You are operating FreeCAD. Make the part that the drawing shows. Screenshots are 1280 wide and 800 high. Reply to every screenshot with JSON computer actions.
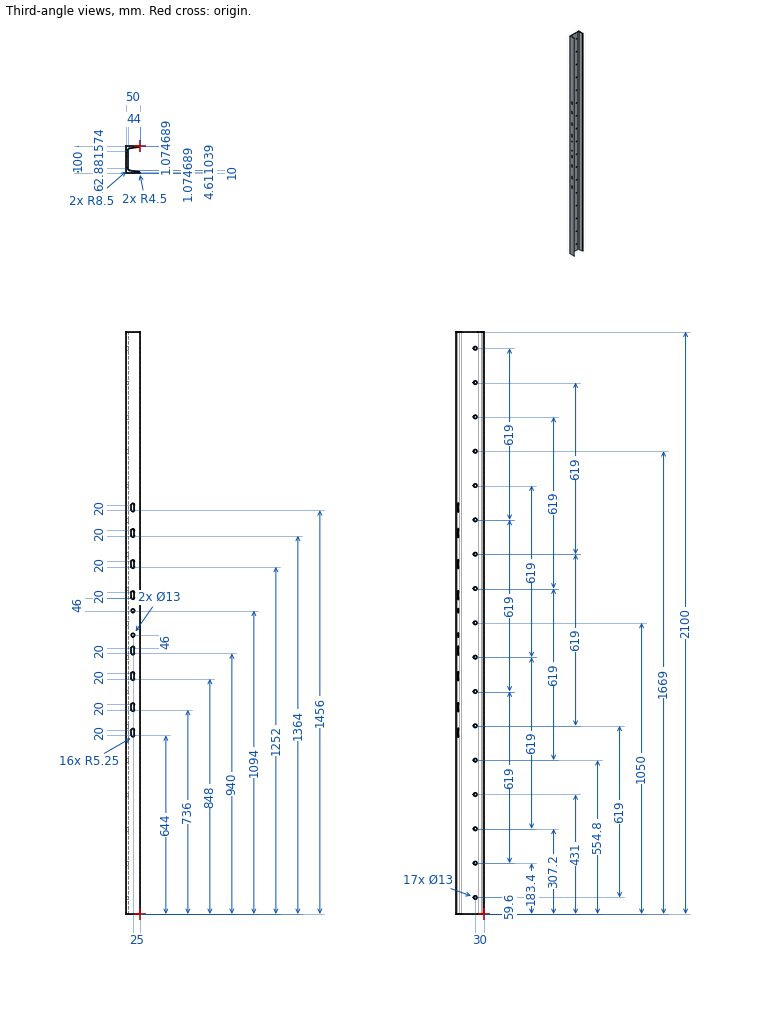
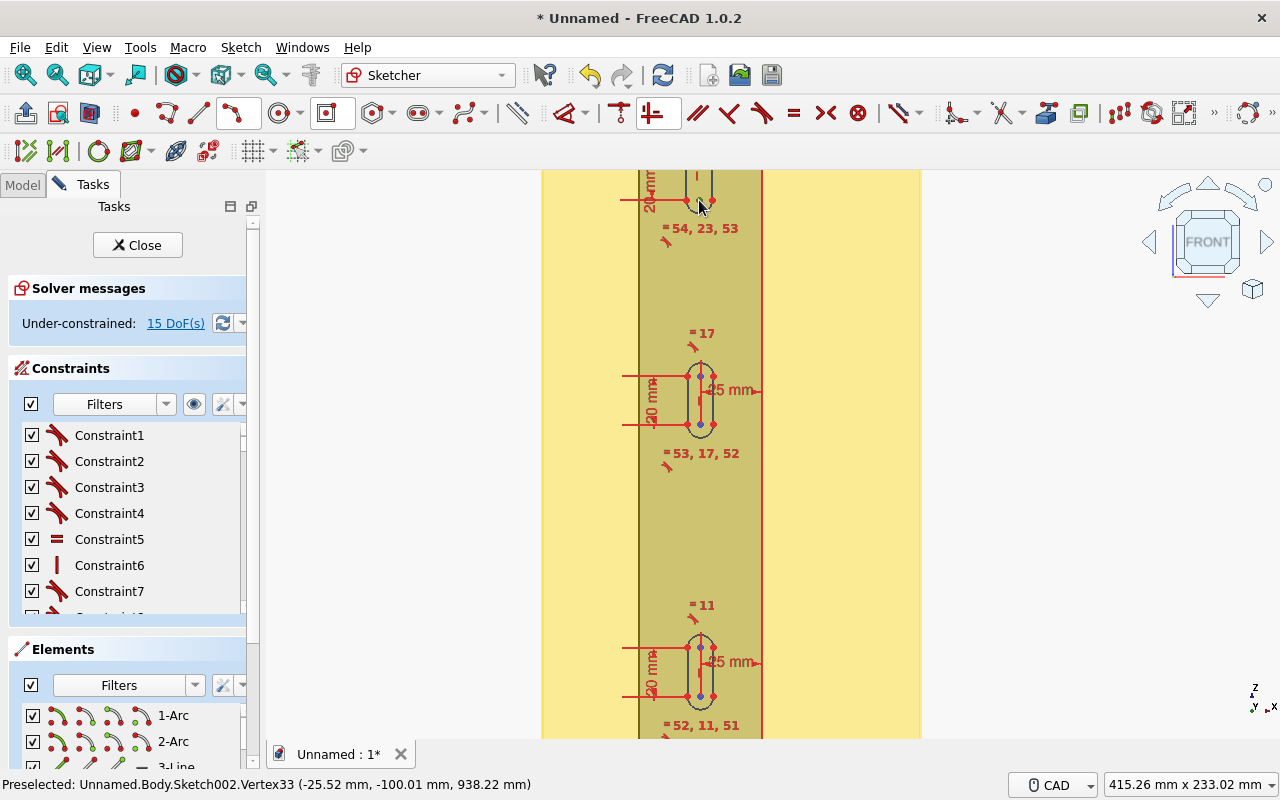
{"action": "left_click", "coordinate": [588, 114]}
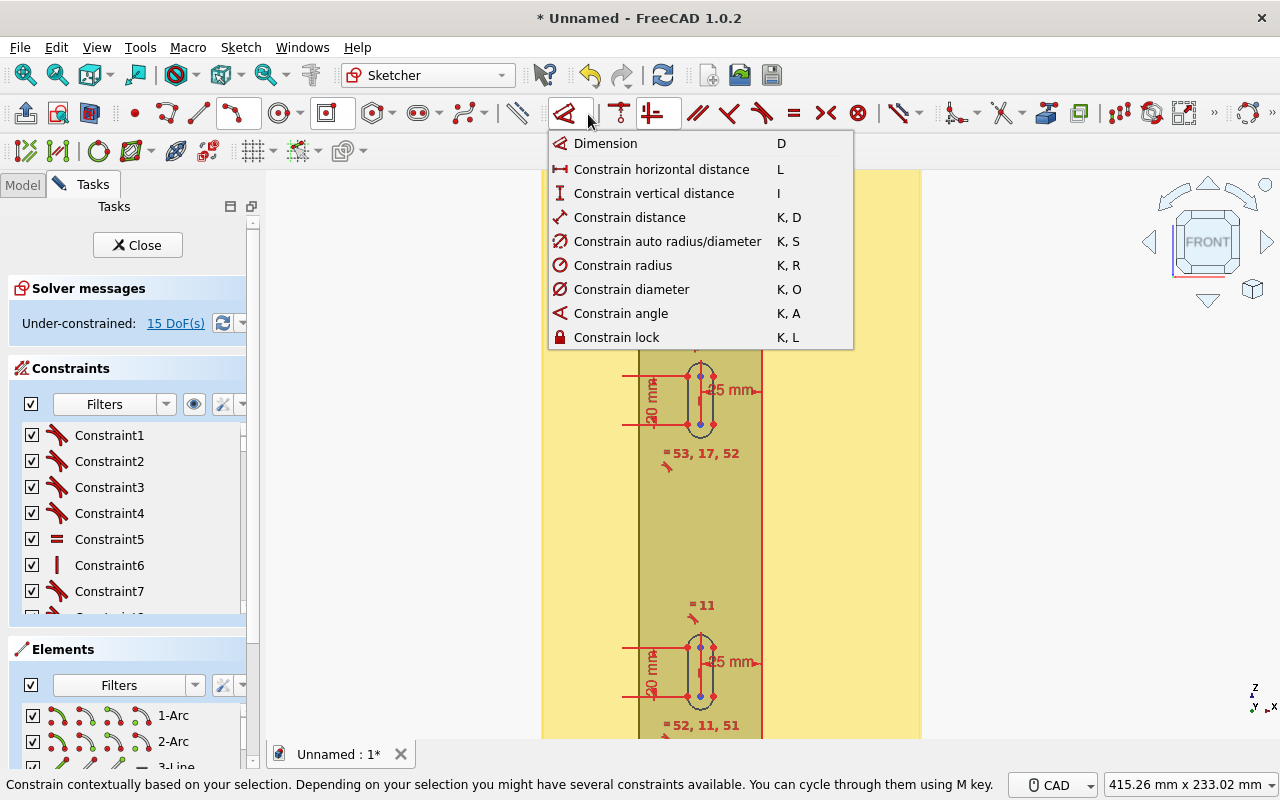
{"action": "left_click", "coordinate": [701, 169]}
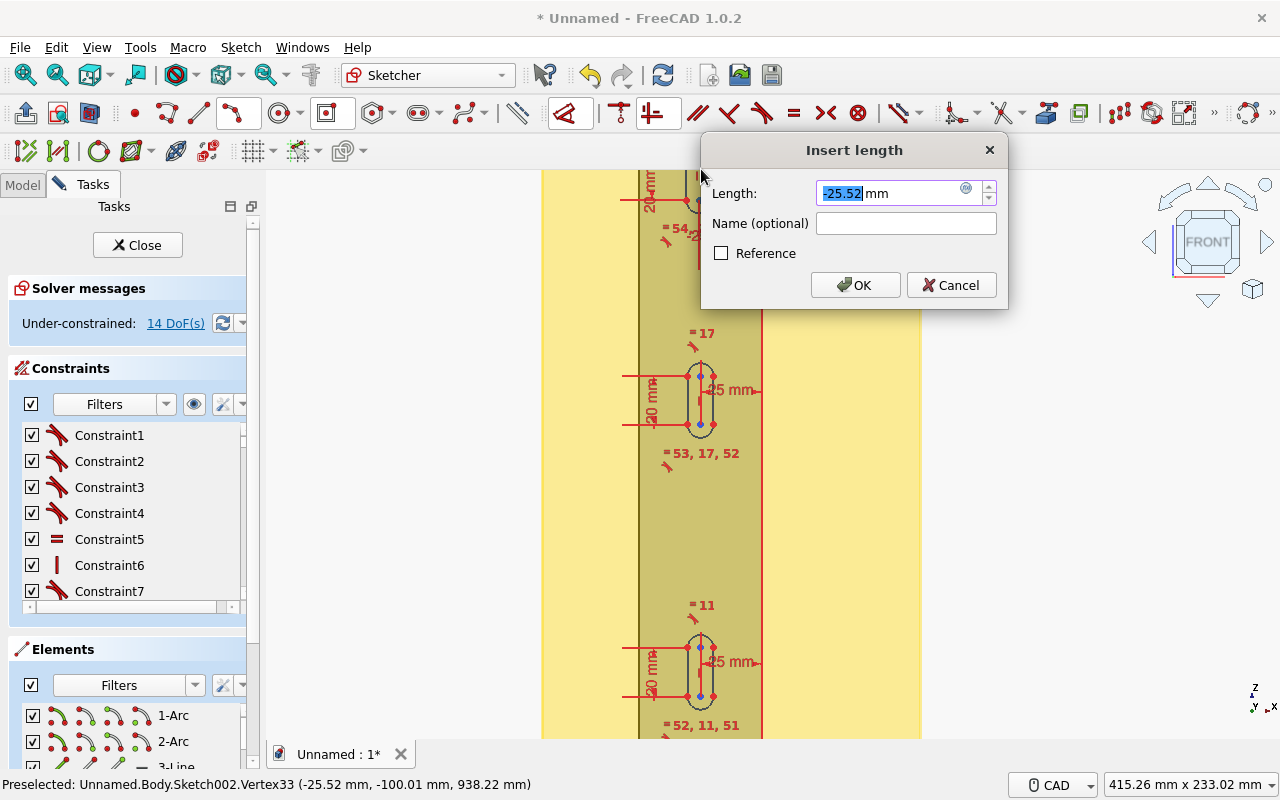
{"action": "type", "text": "-25"}
{"action": "key", "text": "Return"}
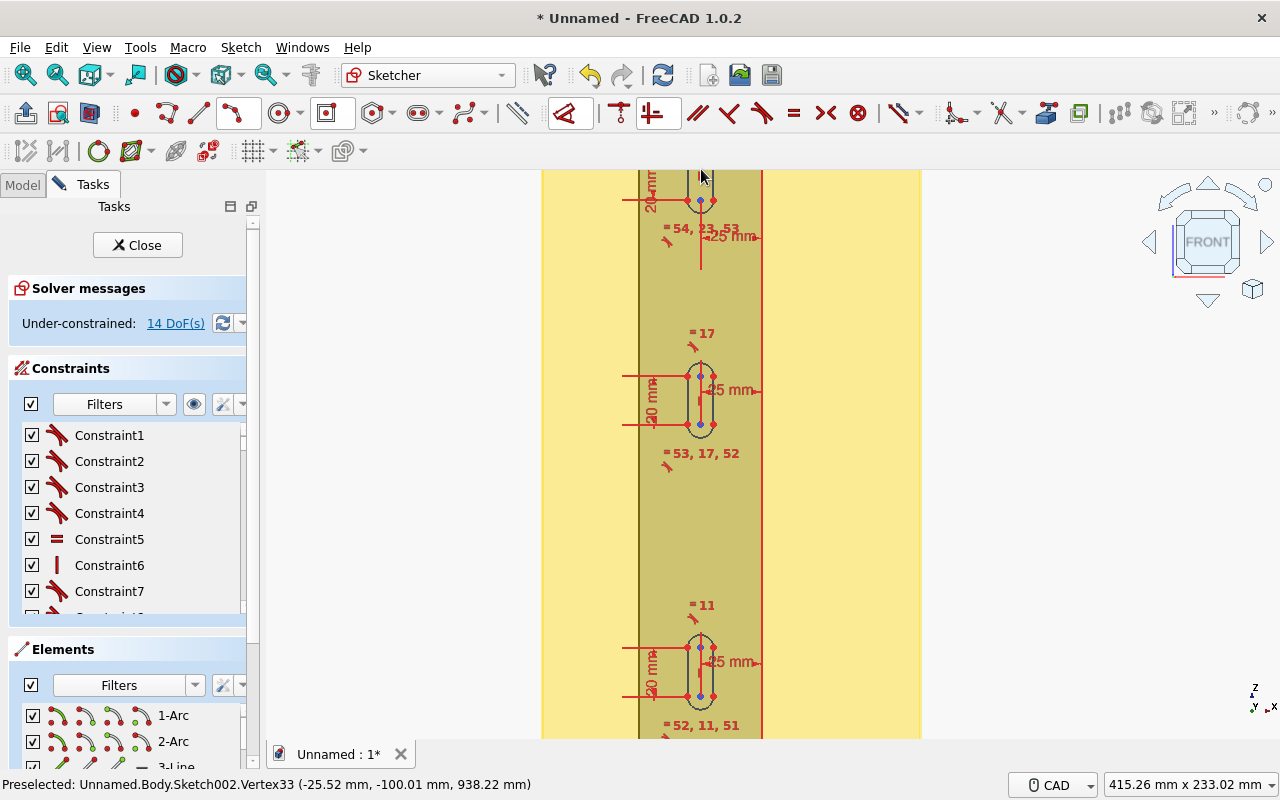
{"action": "scroll", "coordinate": [703, 432], "scroll_direction": "down", "scroll_amount": 12}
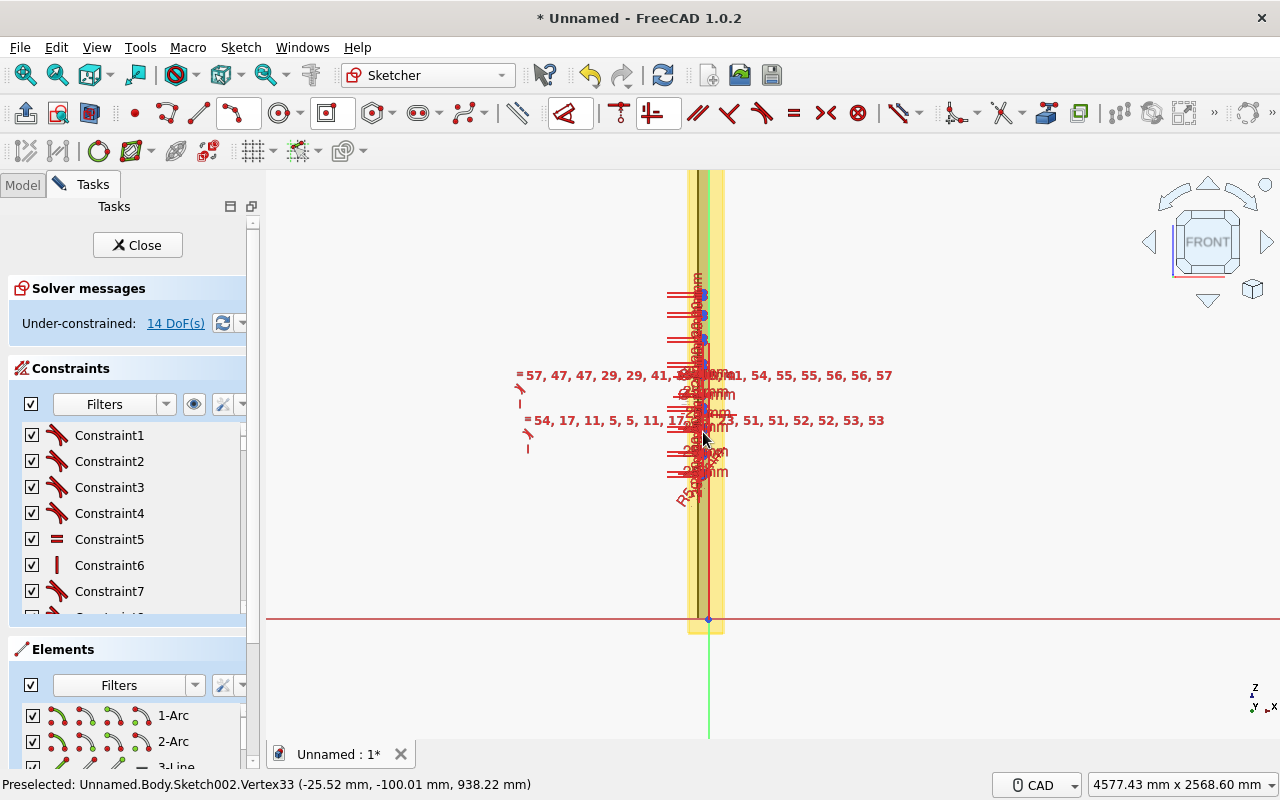
{"action": "scroll", "coordinate": [703, 342], "scroll_direction": "up", "scroll_amount": 12}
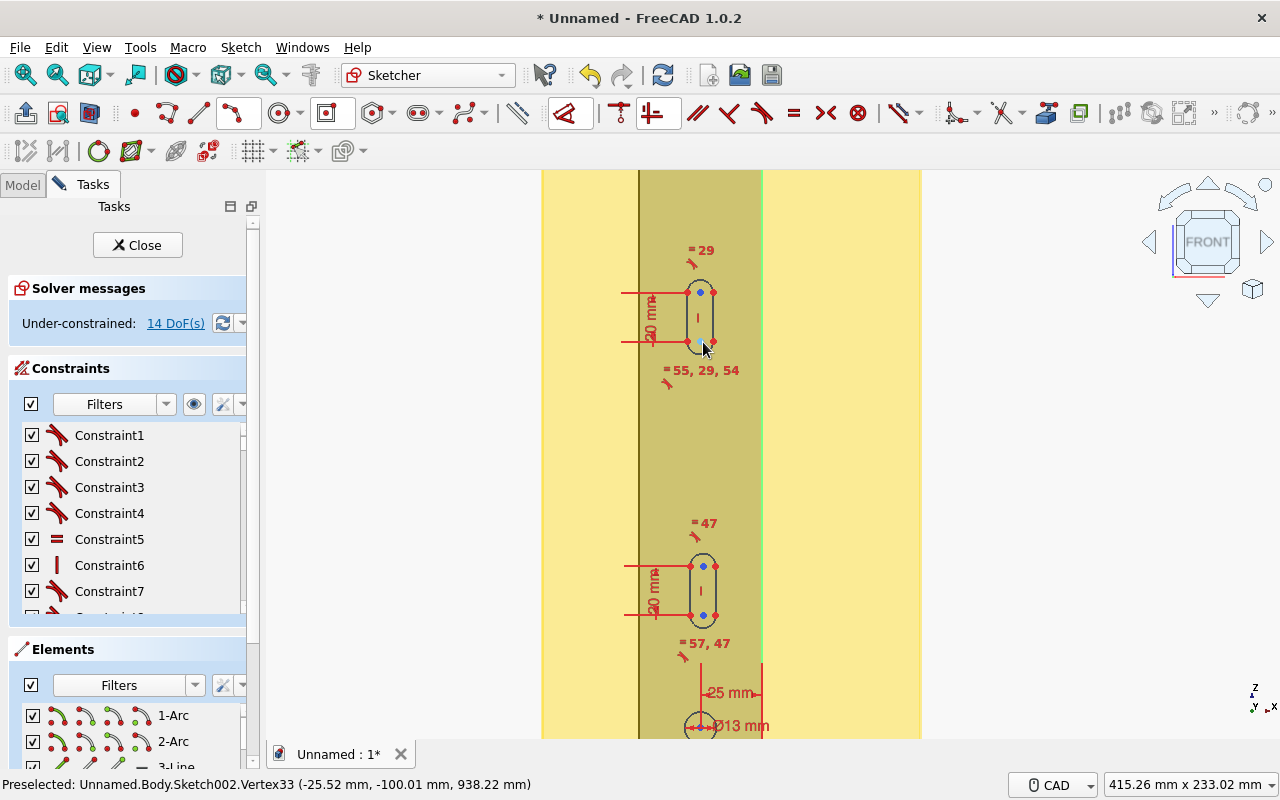
{"action": "left_click", "coordinate": [700, 342]}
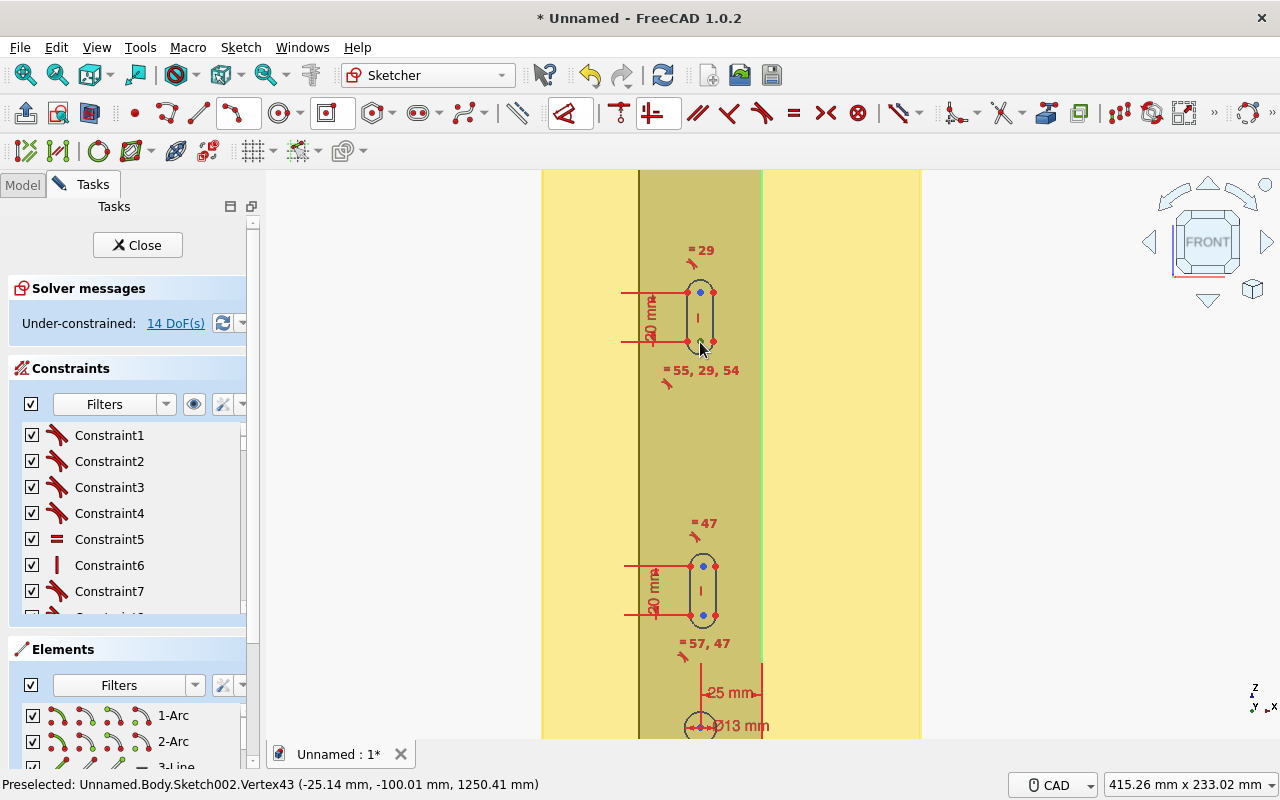
{"action": "left_click", "coordinate": [588, 114]}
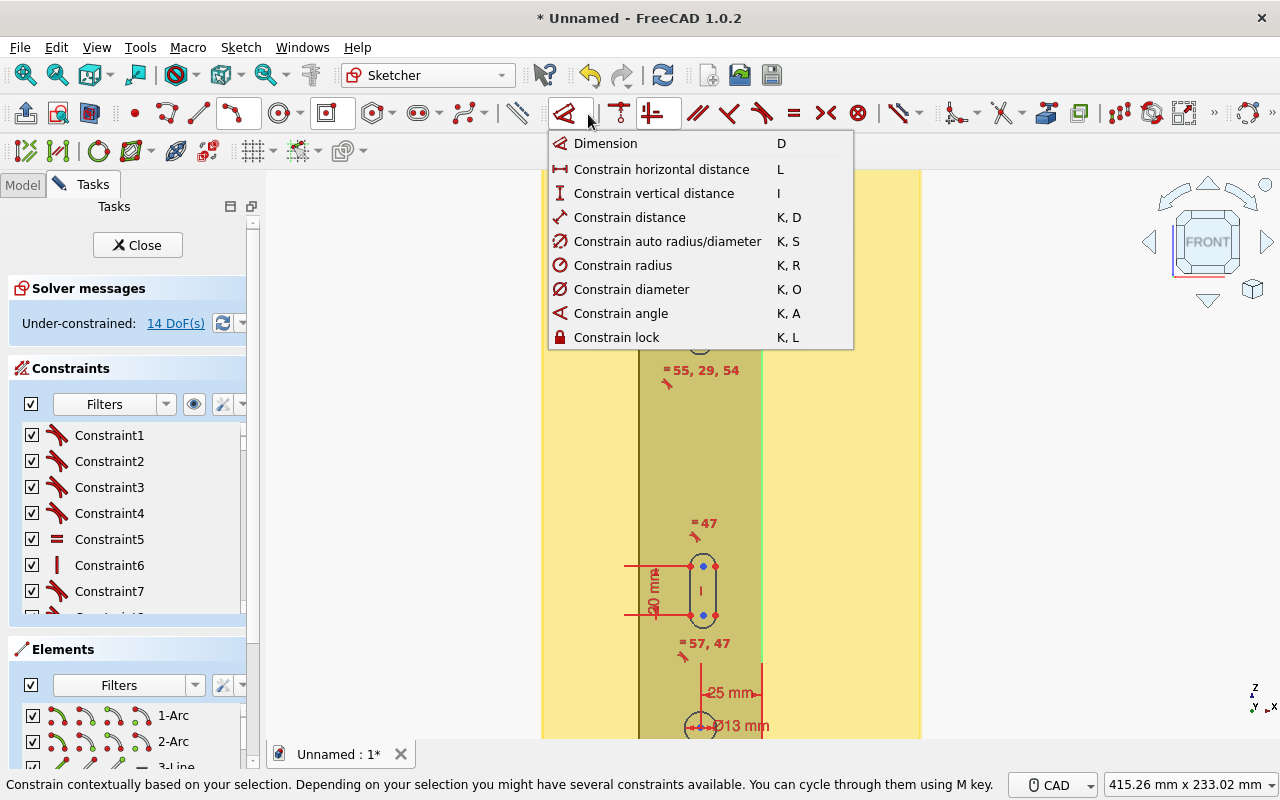
{"action": "left_click", "coordinate": [701, 169]}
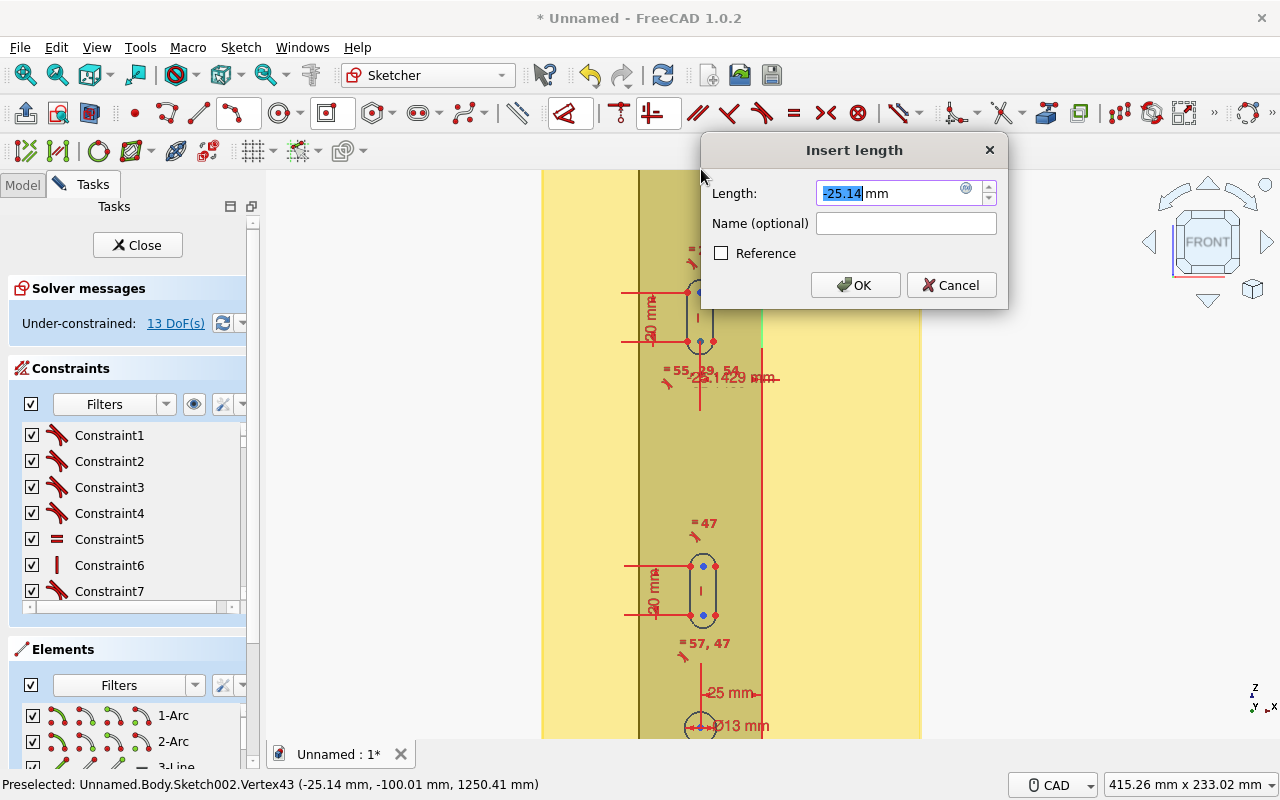
{"action": "type", "text": "-25"}
{"action": "key", "text": "Return"}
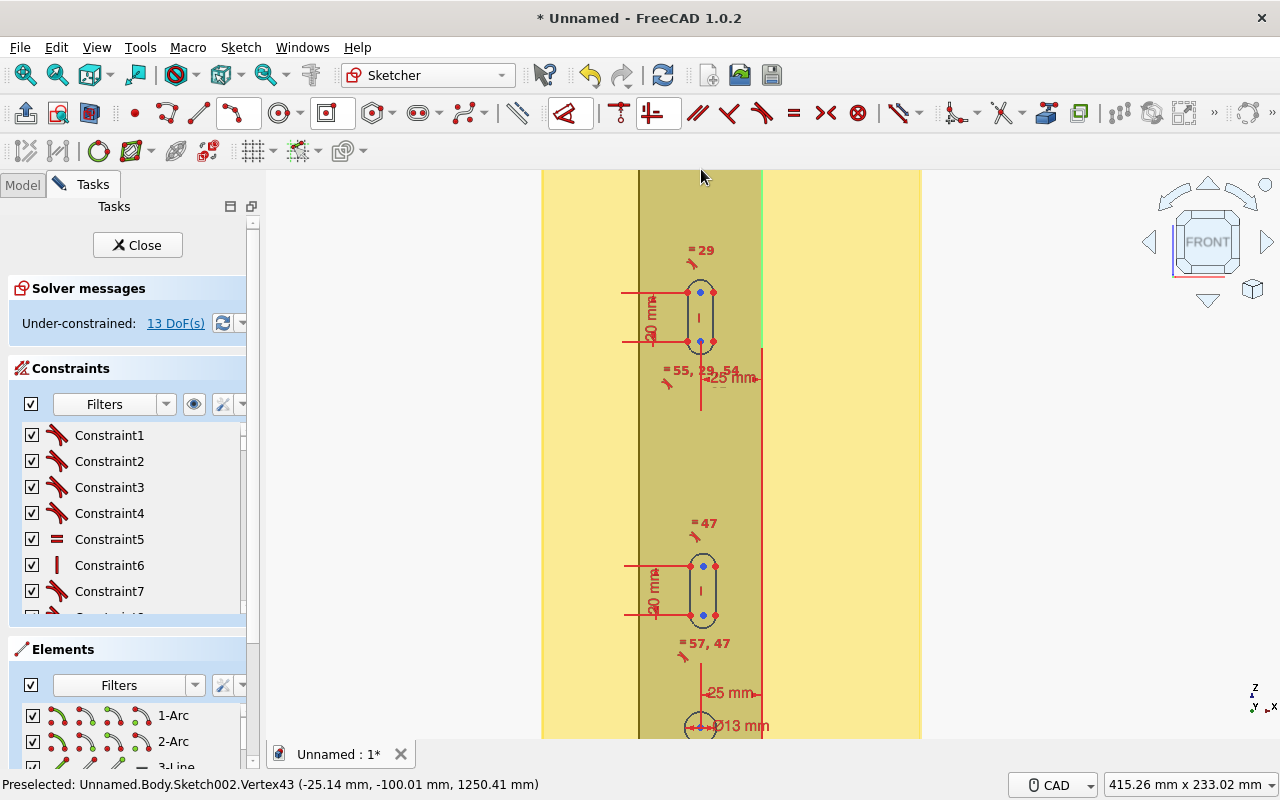
{"action": "scroll", "coordinate": [703, 342], "scroll_direction": "down", "scroll_amount": 12}